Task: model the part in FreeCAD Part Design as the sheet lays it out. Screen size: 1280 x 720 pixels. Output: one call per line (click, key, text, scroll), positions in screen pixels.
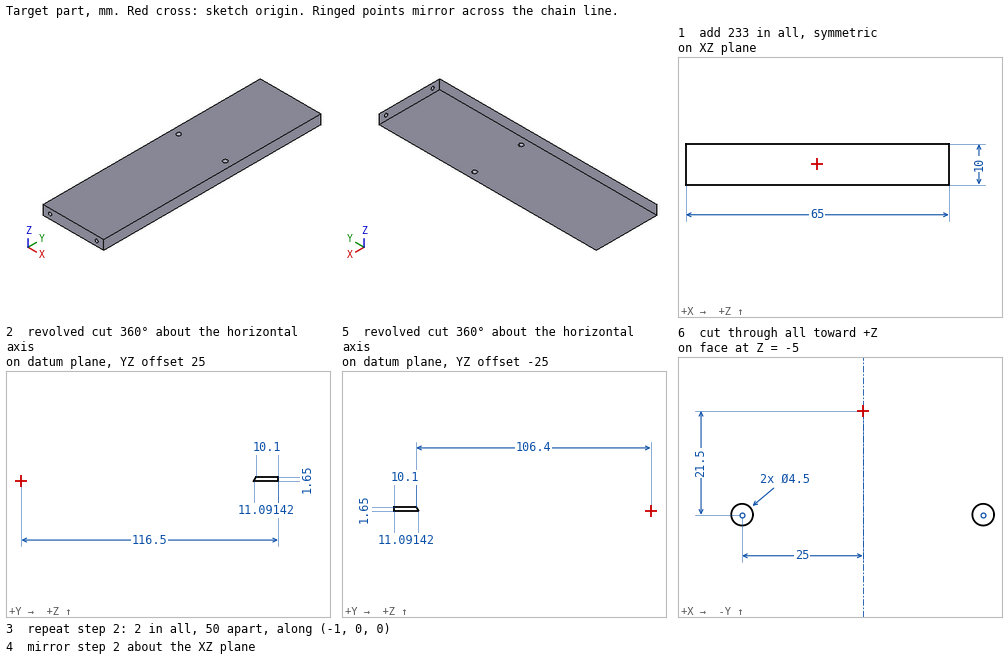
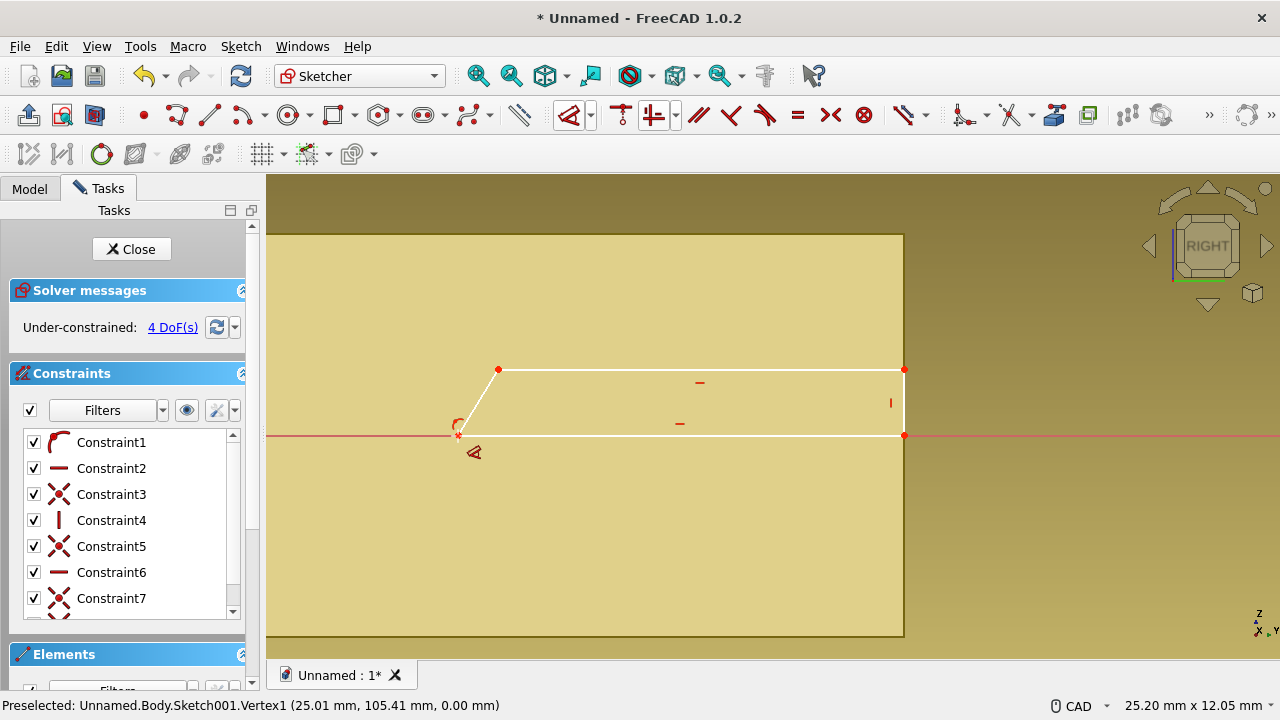
click(904, 416)
click(938, 403)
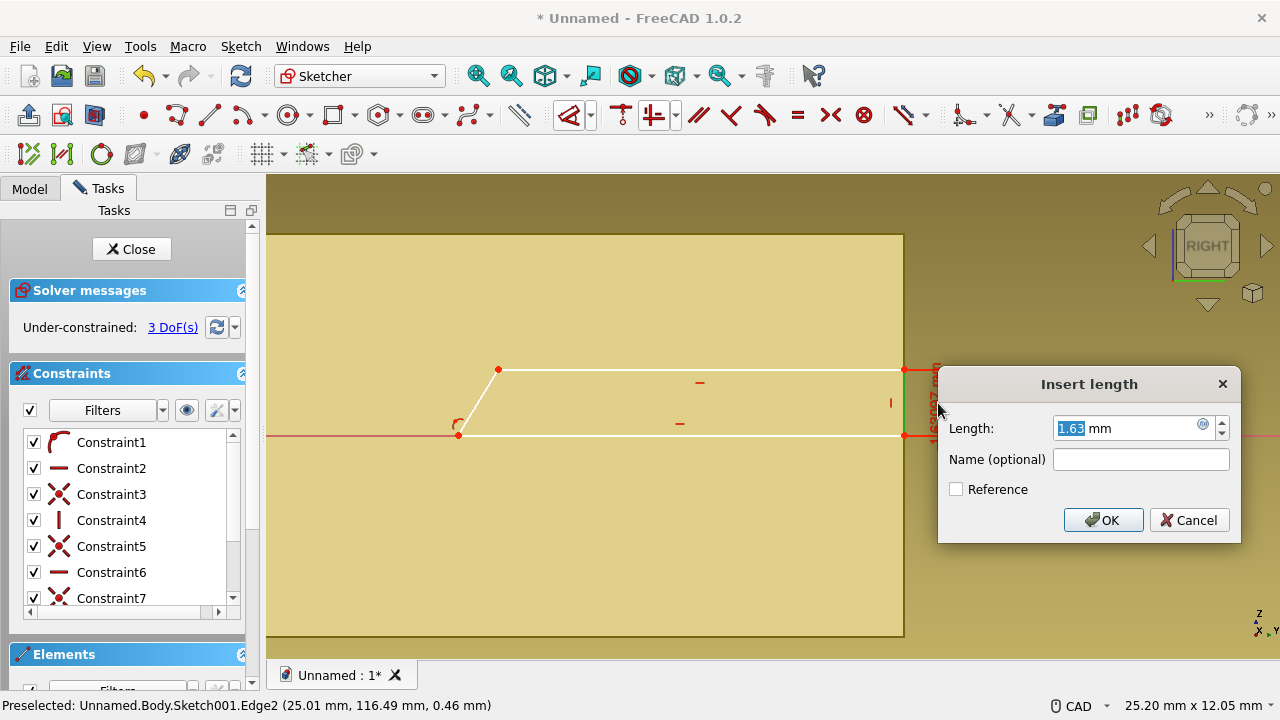
text(1.65)
key(Return)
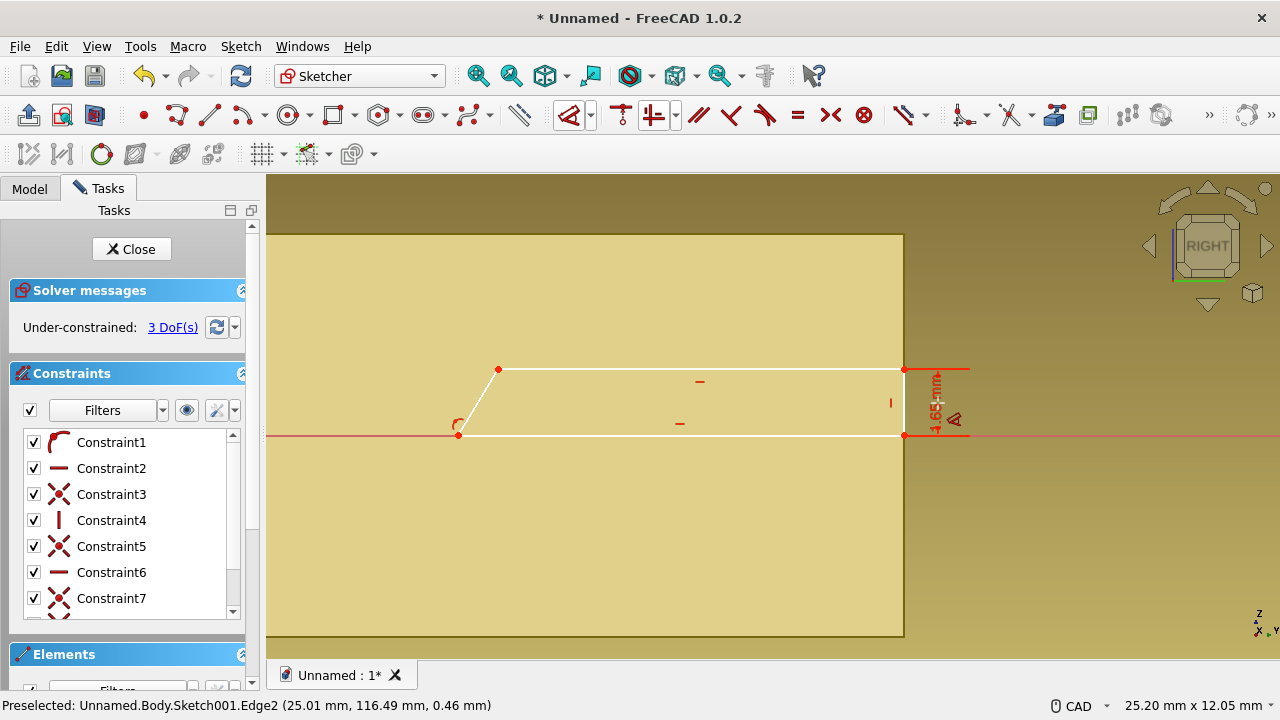
click(782, 369)
click(701, 335)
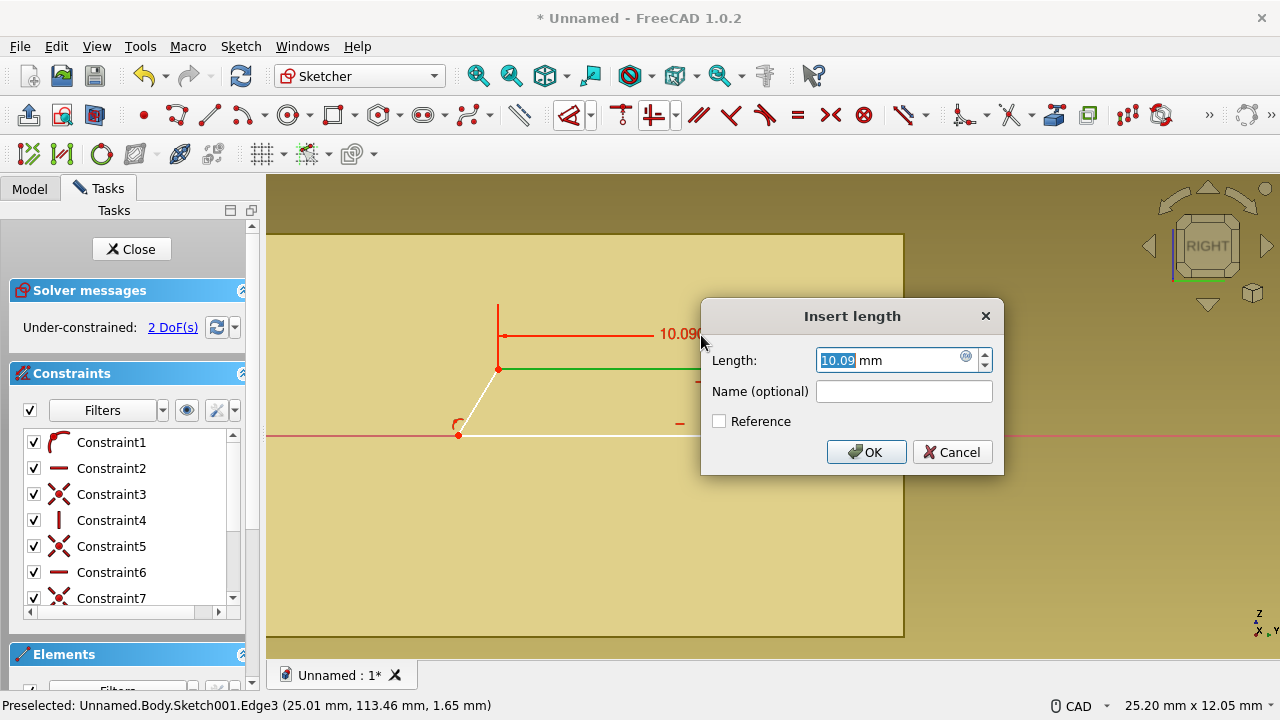
text(10.1)
key(Return)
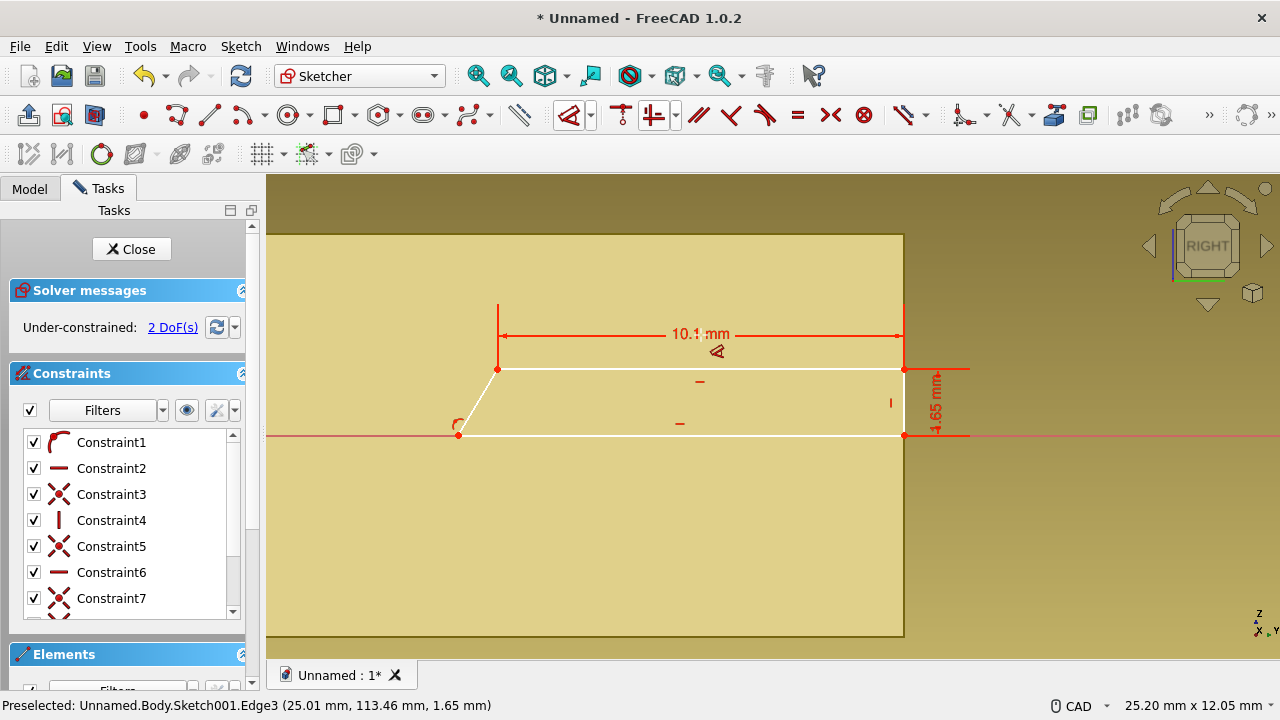
click(904, 436)
click(599, 470)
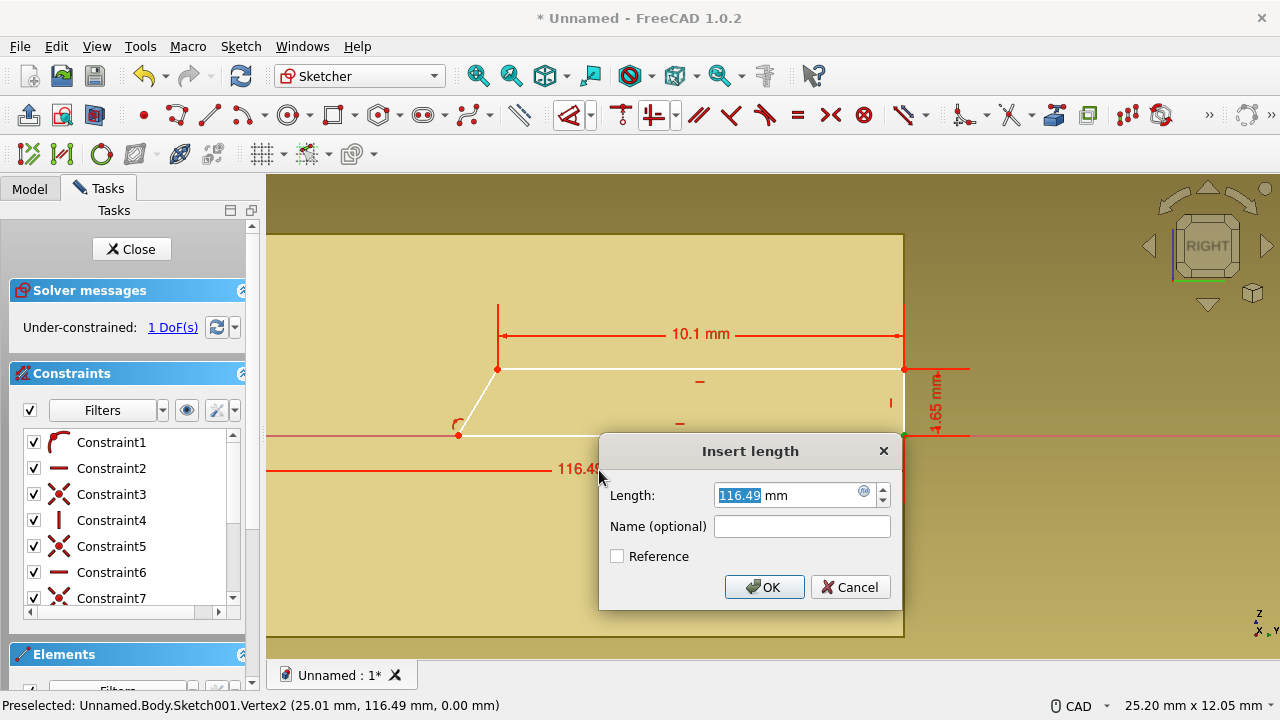
text(116.5)
key(Return)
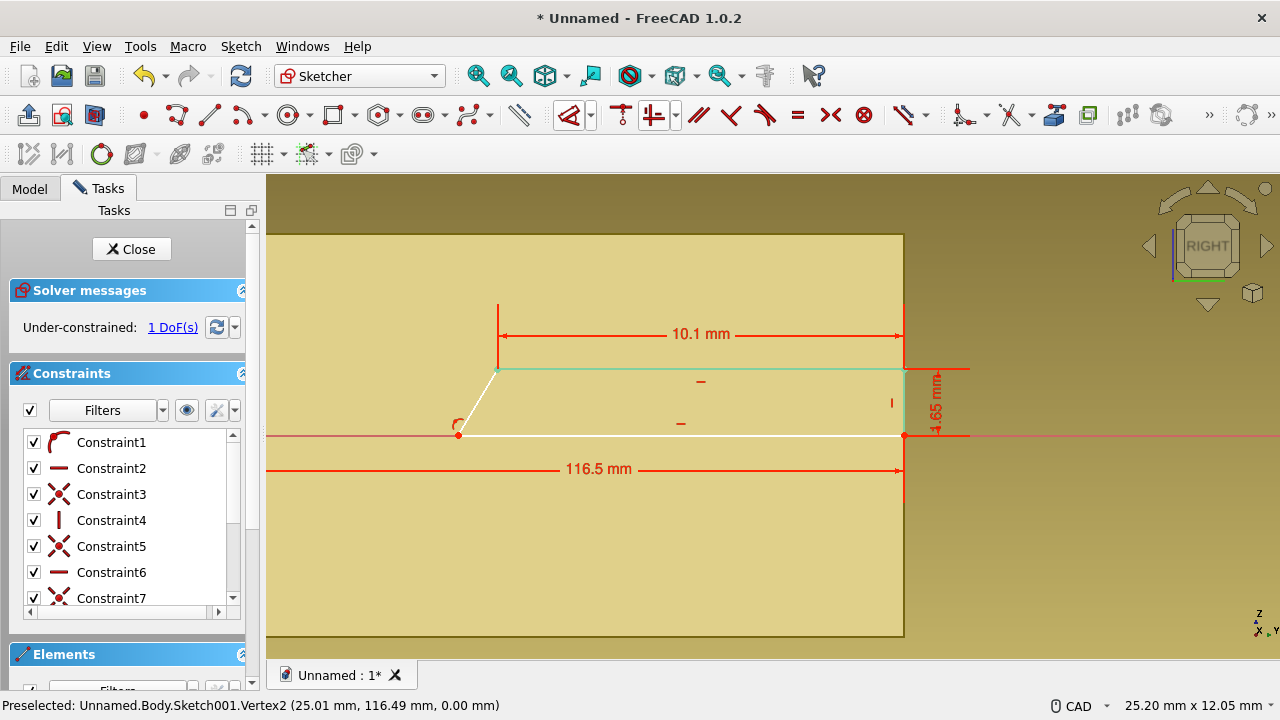
click(592, 436)
click(681, 470)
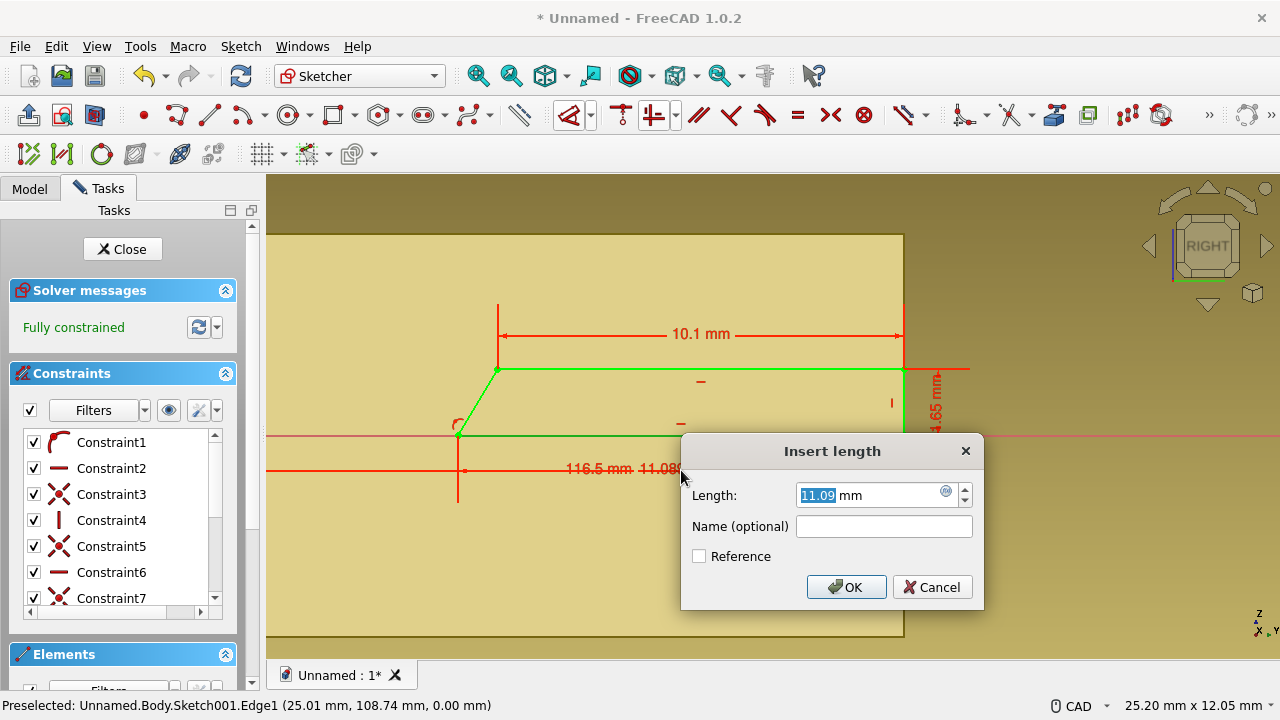
text(11.09142)
key(Return)
key(Escape)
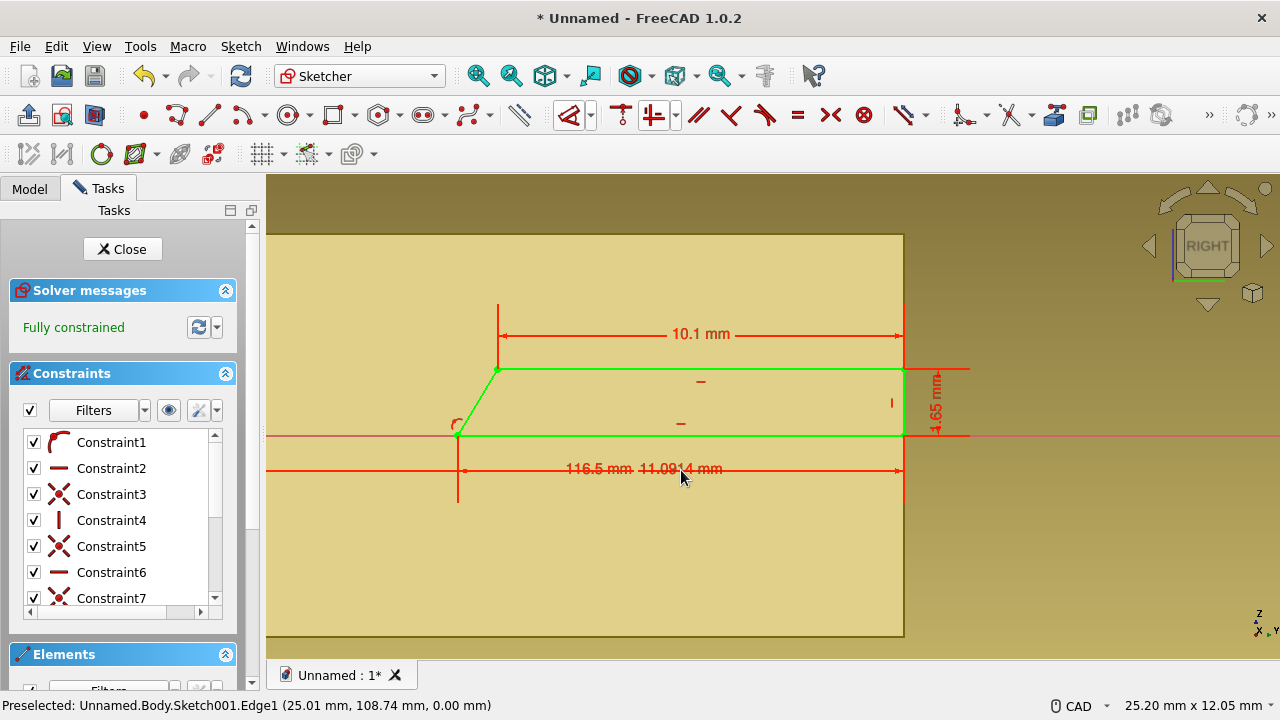
click(123, 249)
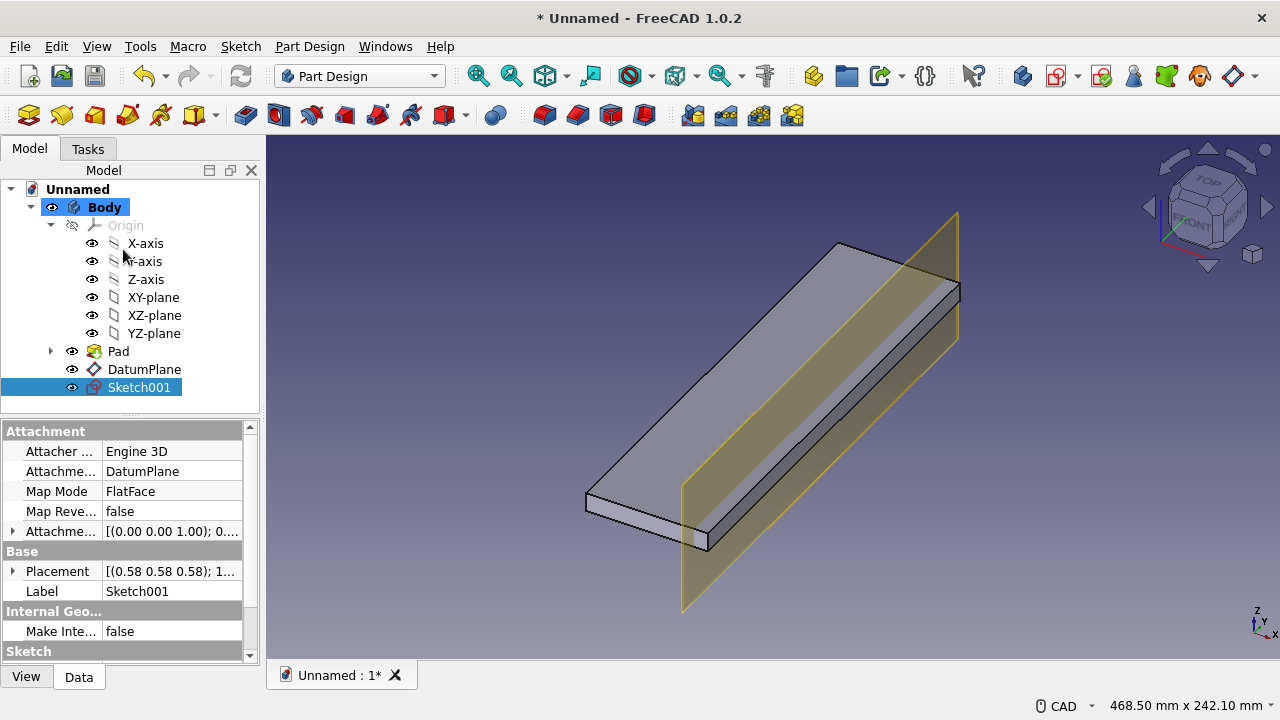
click(312, 116)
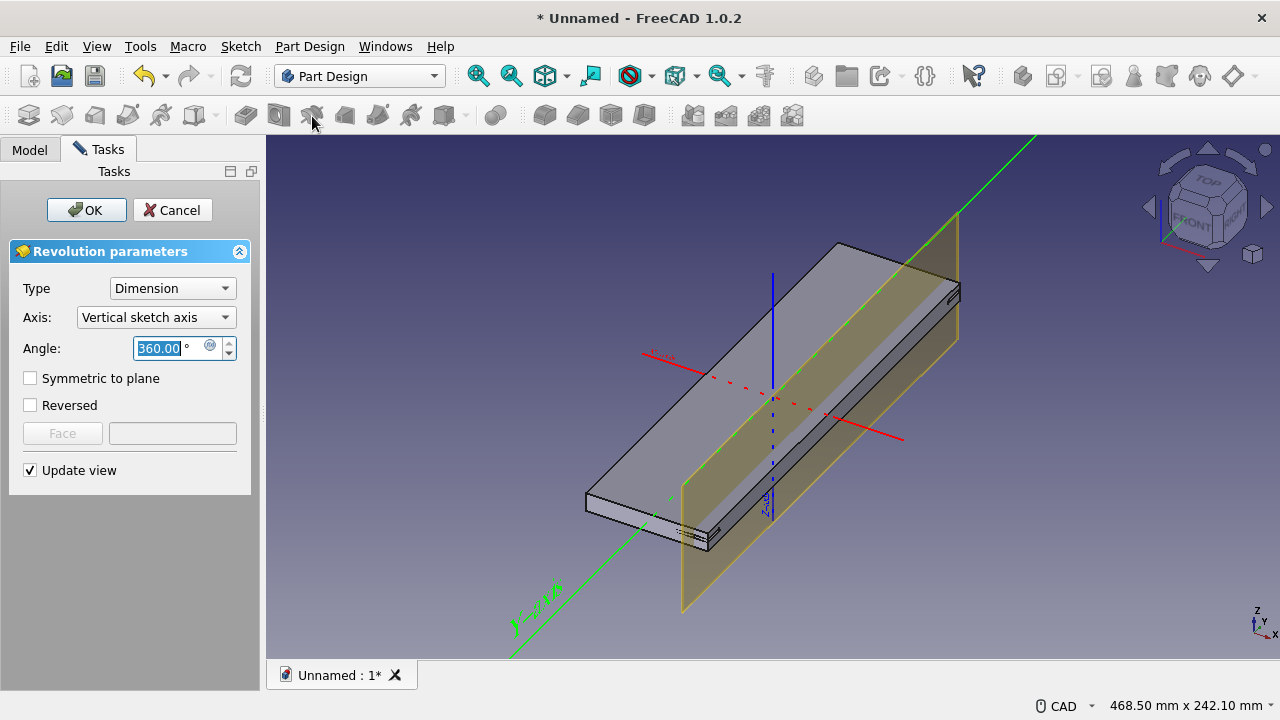
click(157, 318)